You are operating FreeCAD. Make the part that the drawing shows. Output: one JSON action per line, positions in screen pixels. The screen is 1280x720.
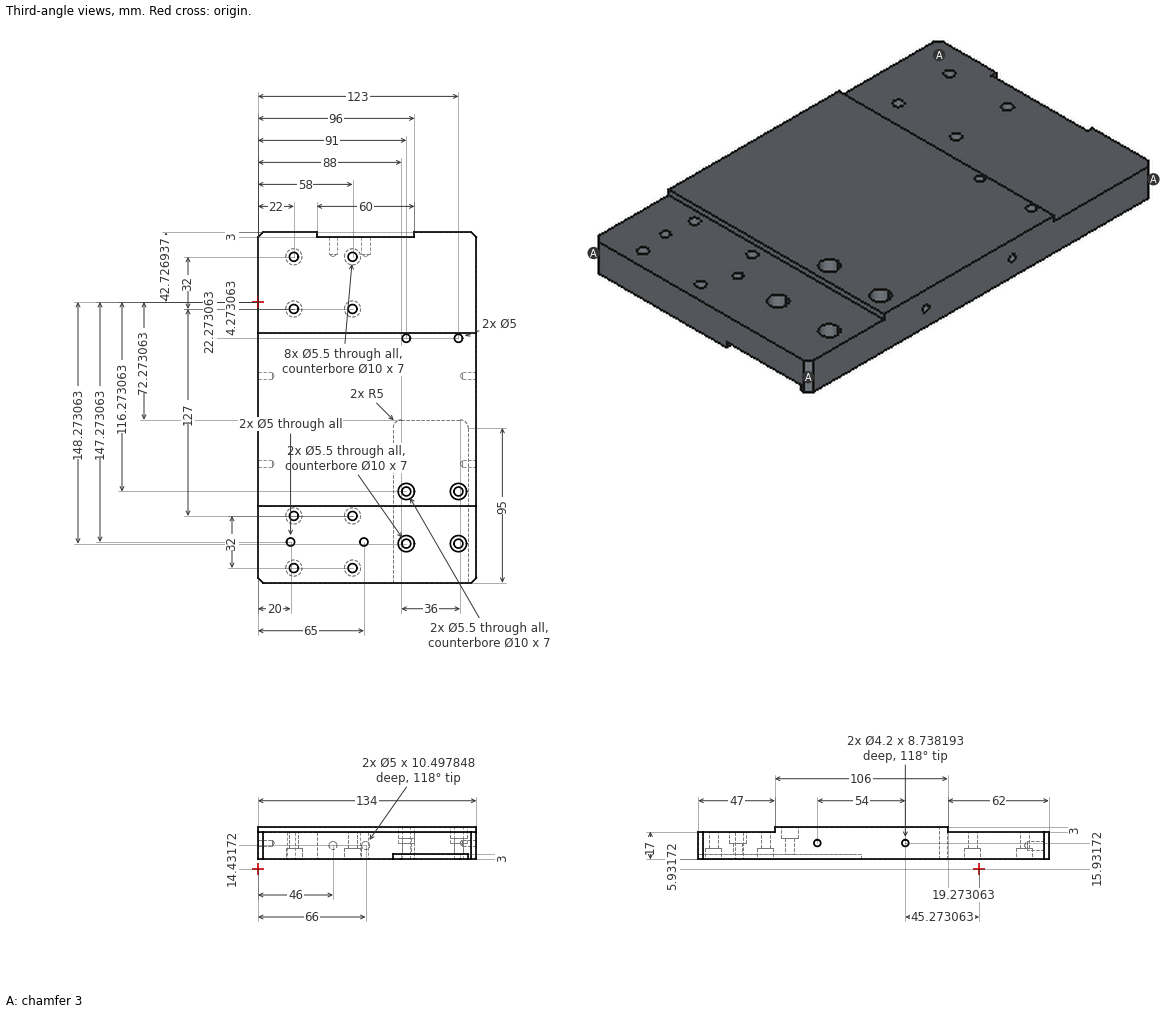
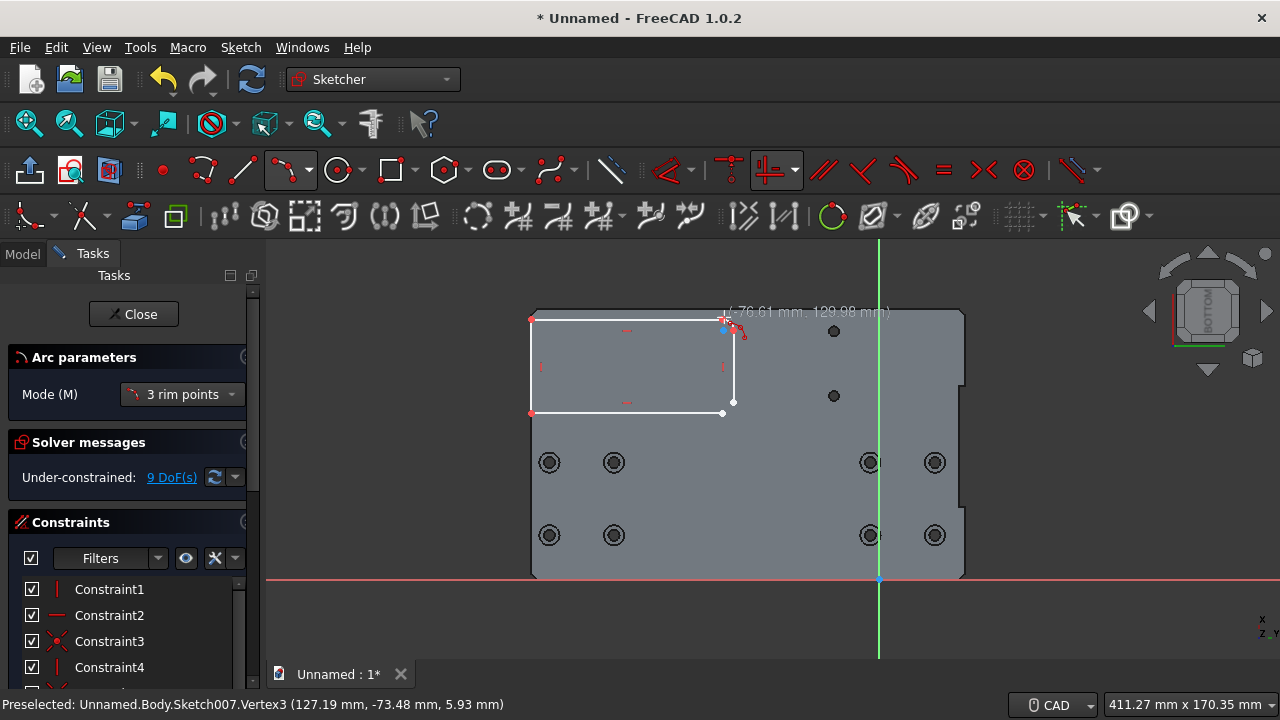
{"action": "left_click", "coordinate": [723, 413]}
{"action": "left_click", "coordinate": [734, 403]}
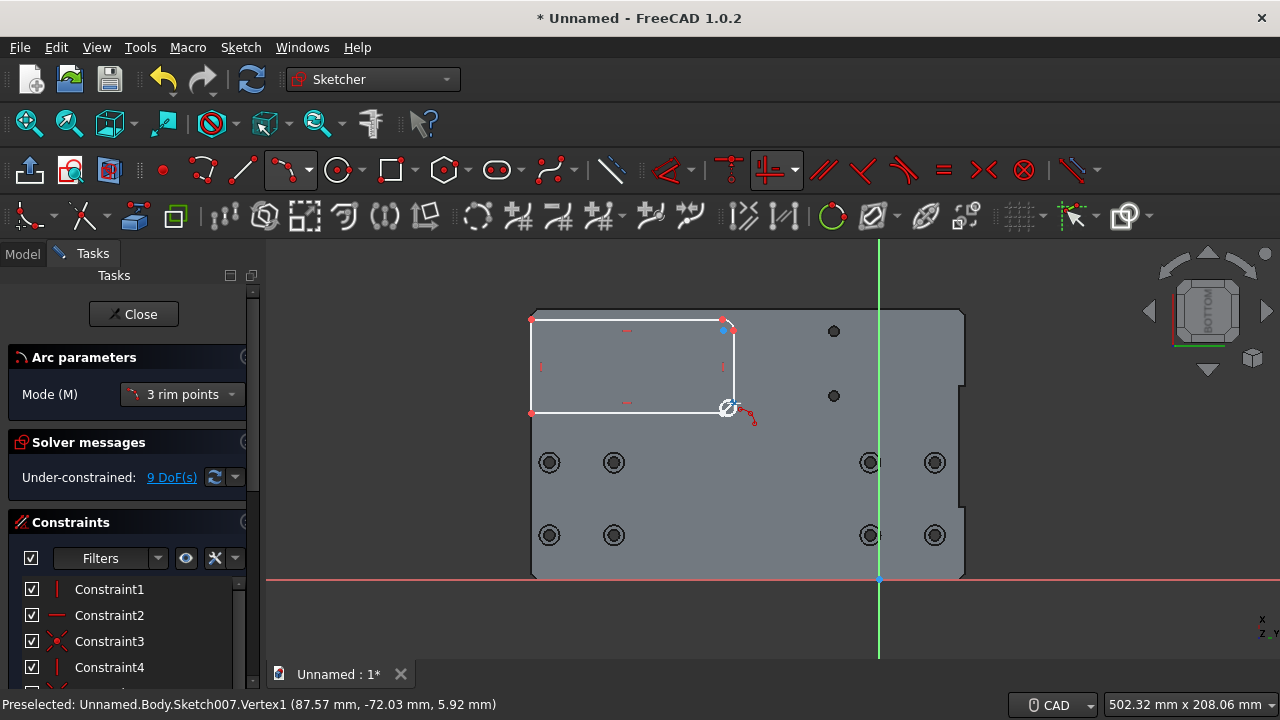
{"action": "scroll", "coordinate": [730, 409], "scroll_direction": "up", "scroll_amount": 9}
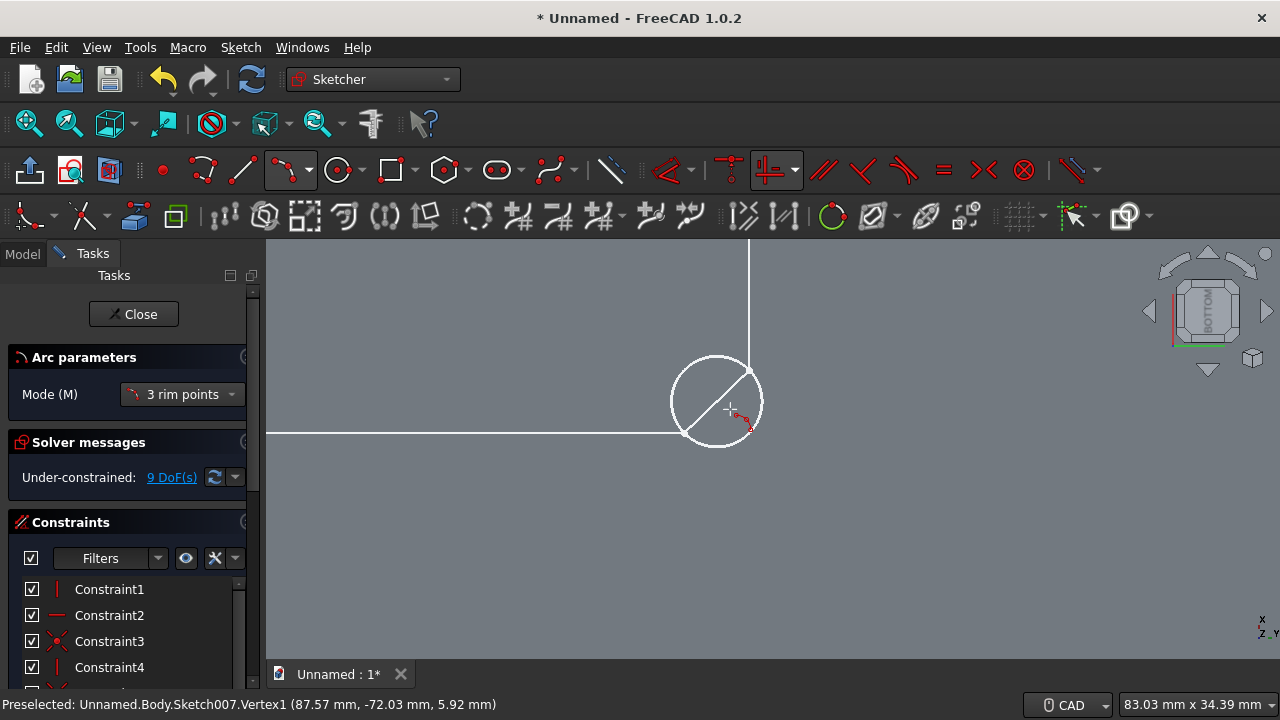
{"action": "left_click", "coordinate": [729, 408]}
{"action": "key", "text": "Escape"}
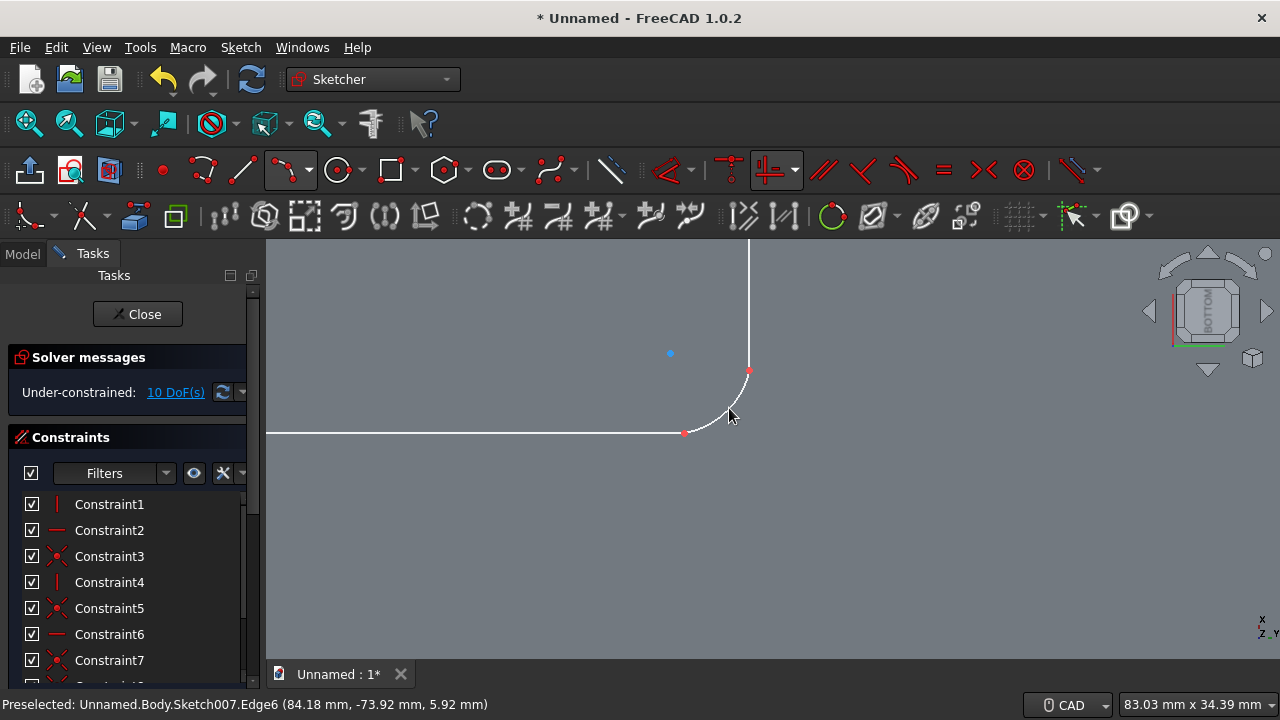
{"action": "scroll", "coordinate": [730, 409], "scroll_direction": "down", "scroll_amount": 9}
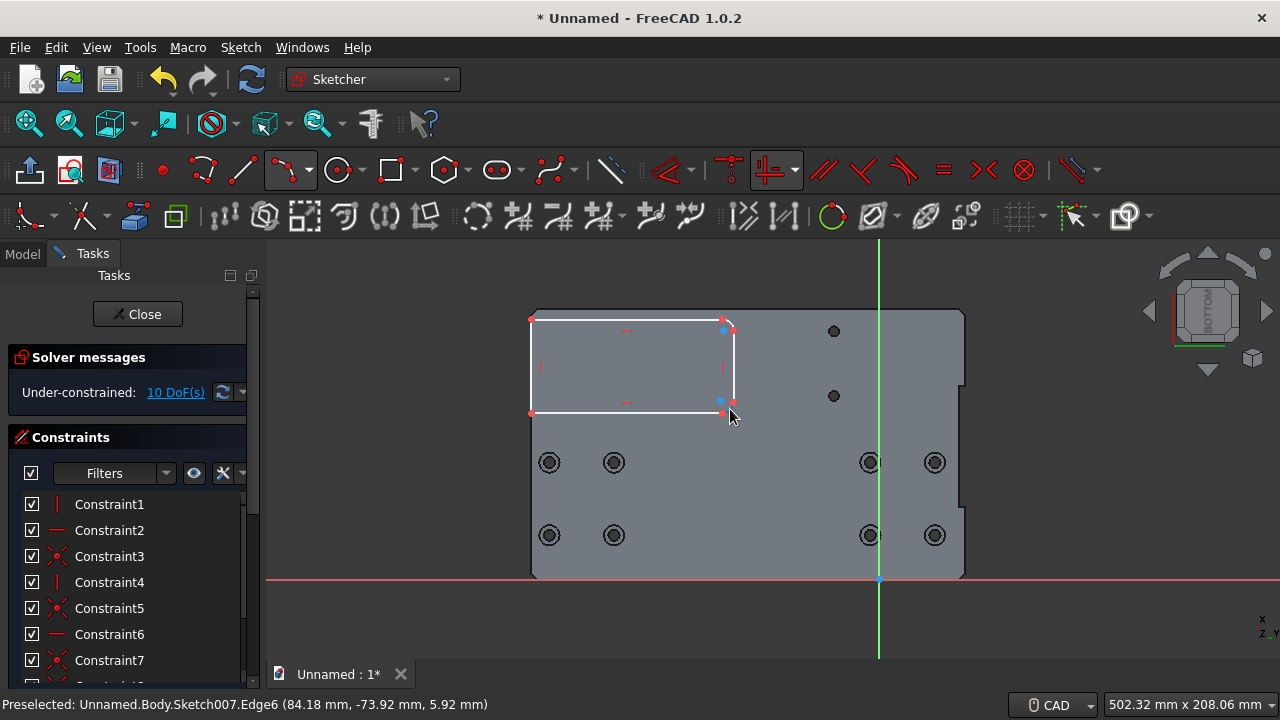
{"action": "left_click", "coordinate": [734, 389]}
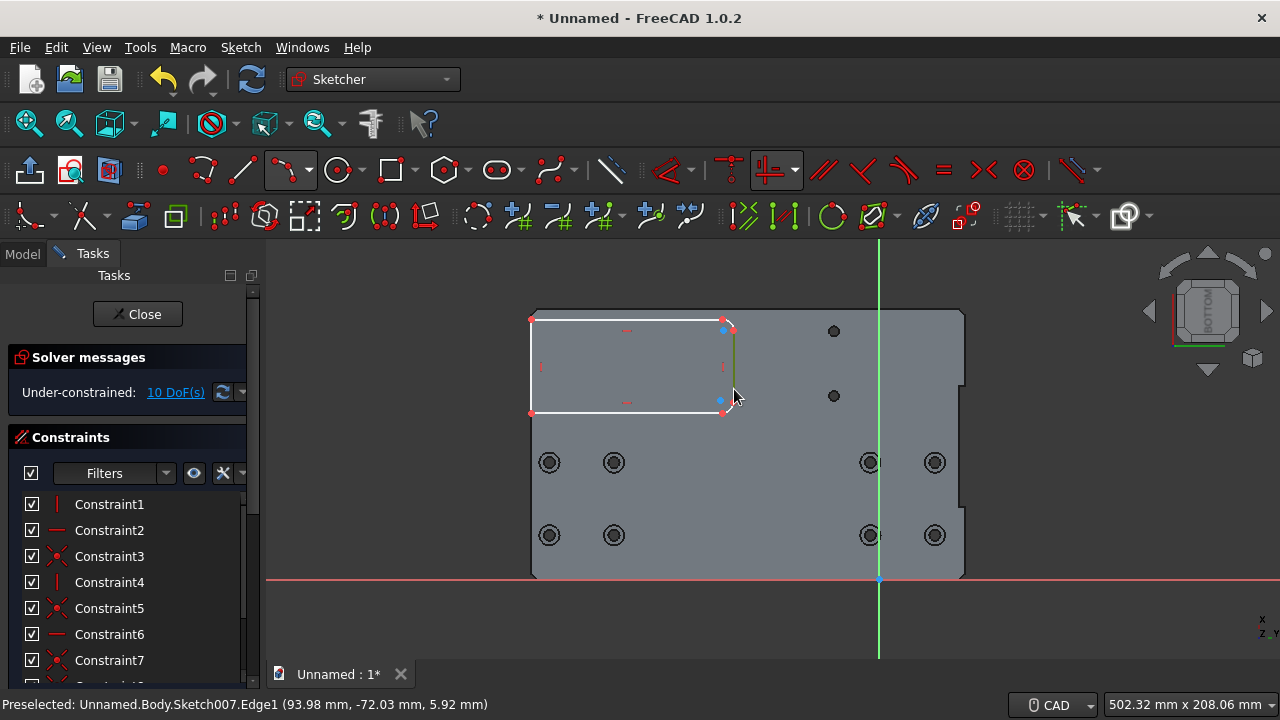
{"action": "scroll", "coordinate": [731, 323], "scroll_direction": "up", "scroll_amount": 3}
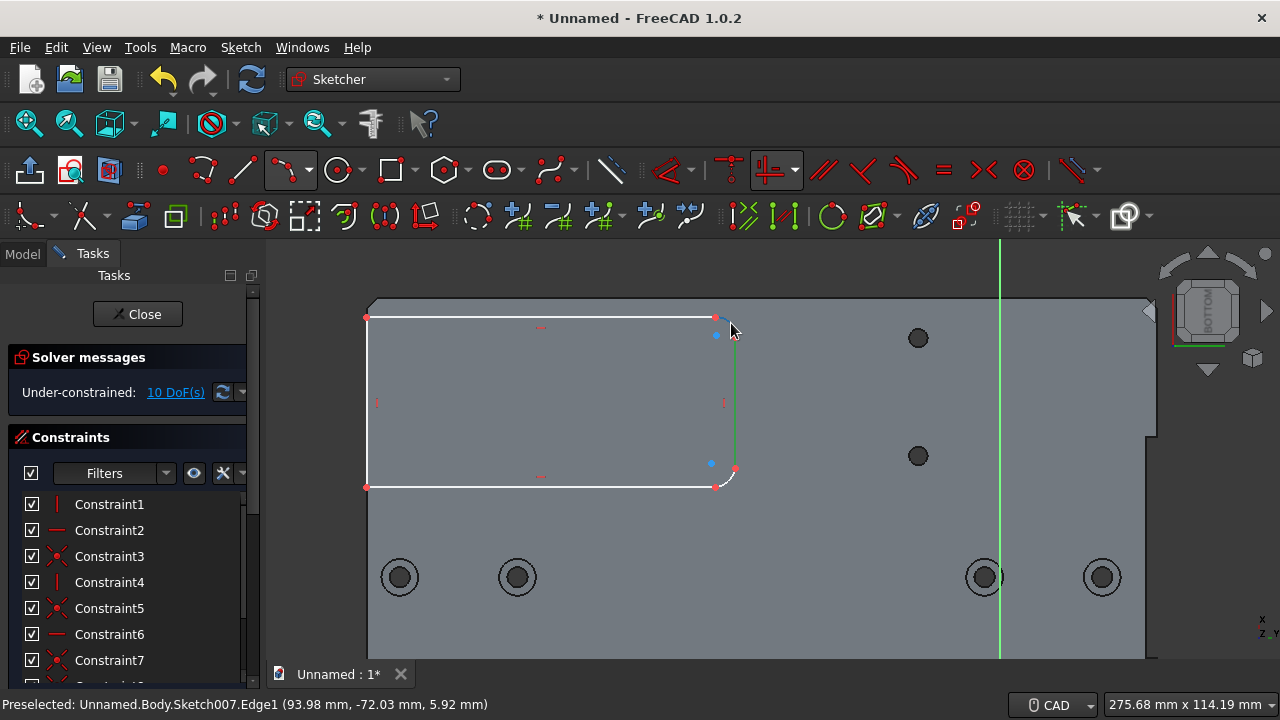
{"action": "left_click", "coordinate": [730, 323]}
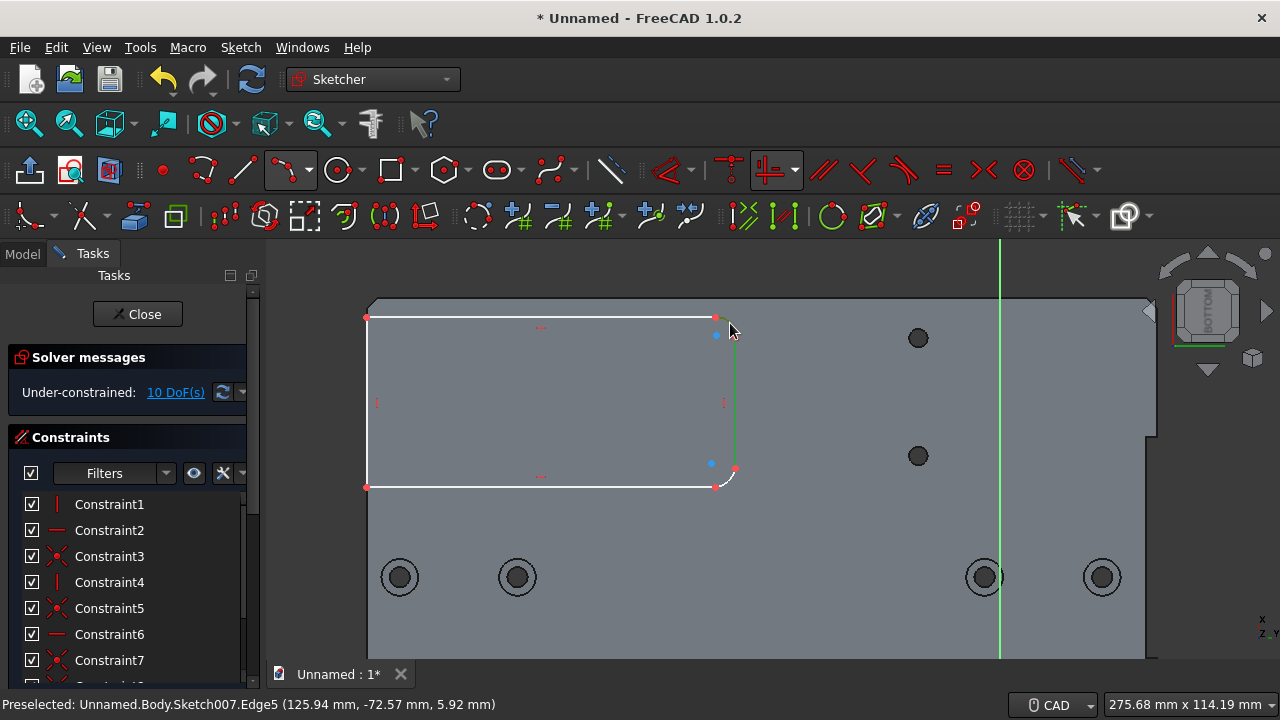
{"action": "left_click", "coordinate": [904, 170]}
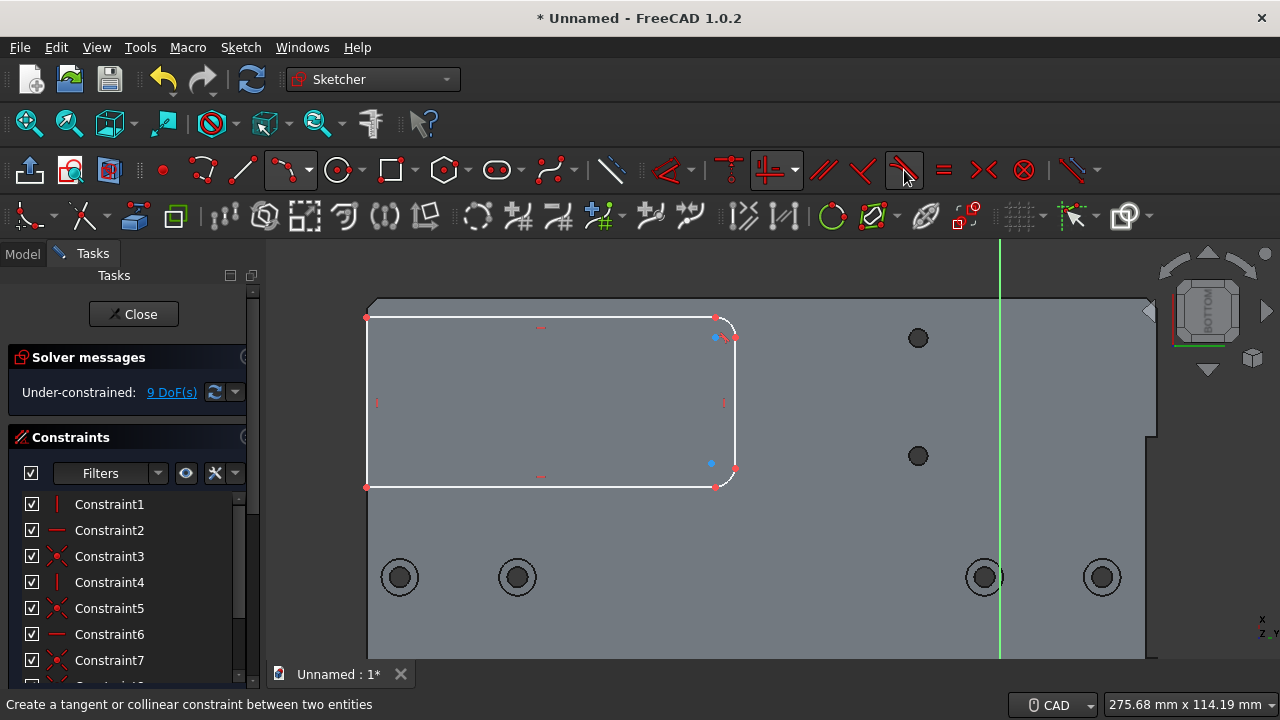
{"action": "left_click", "coordinate": [735, 429]}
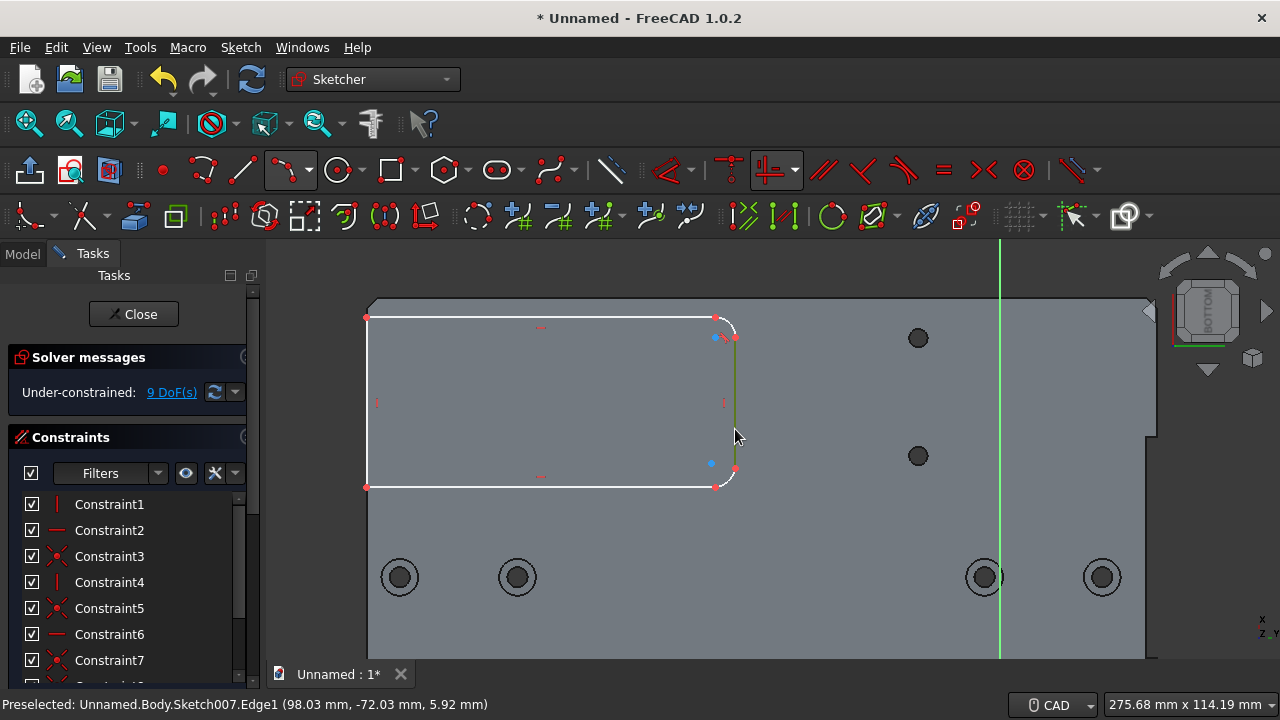
{"action": "left_click", "coordinate": [728, 481]}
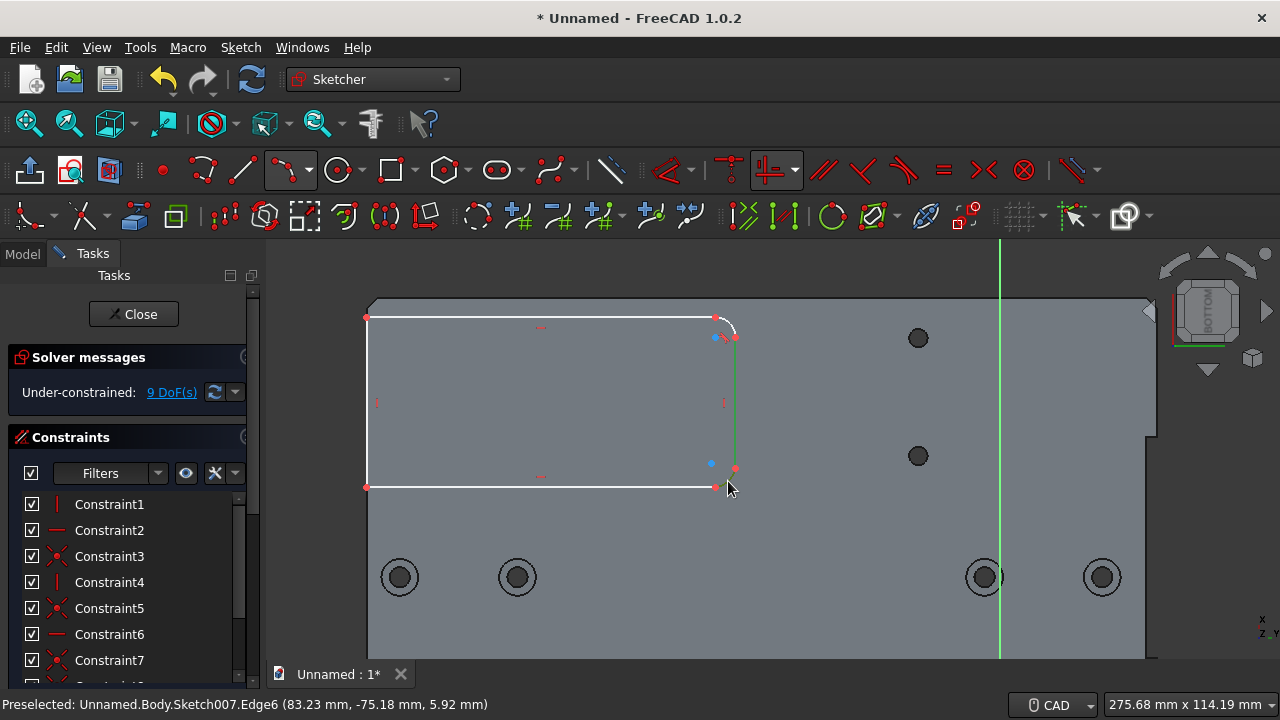
{"action": "left_click", "coordinate": [904, 170]}